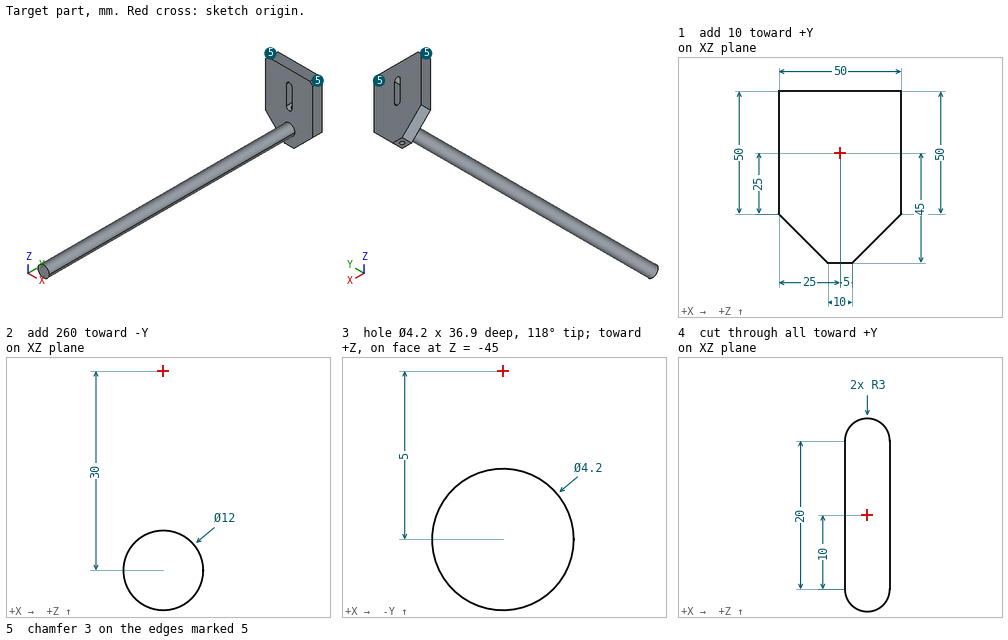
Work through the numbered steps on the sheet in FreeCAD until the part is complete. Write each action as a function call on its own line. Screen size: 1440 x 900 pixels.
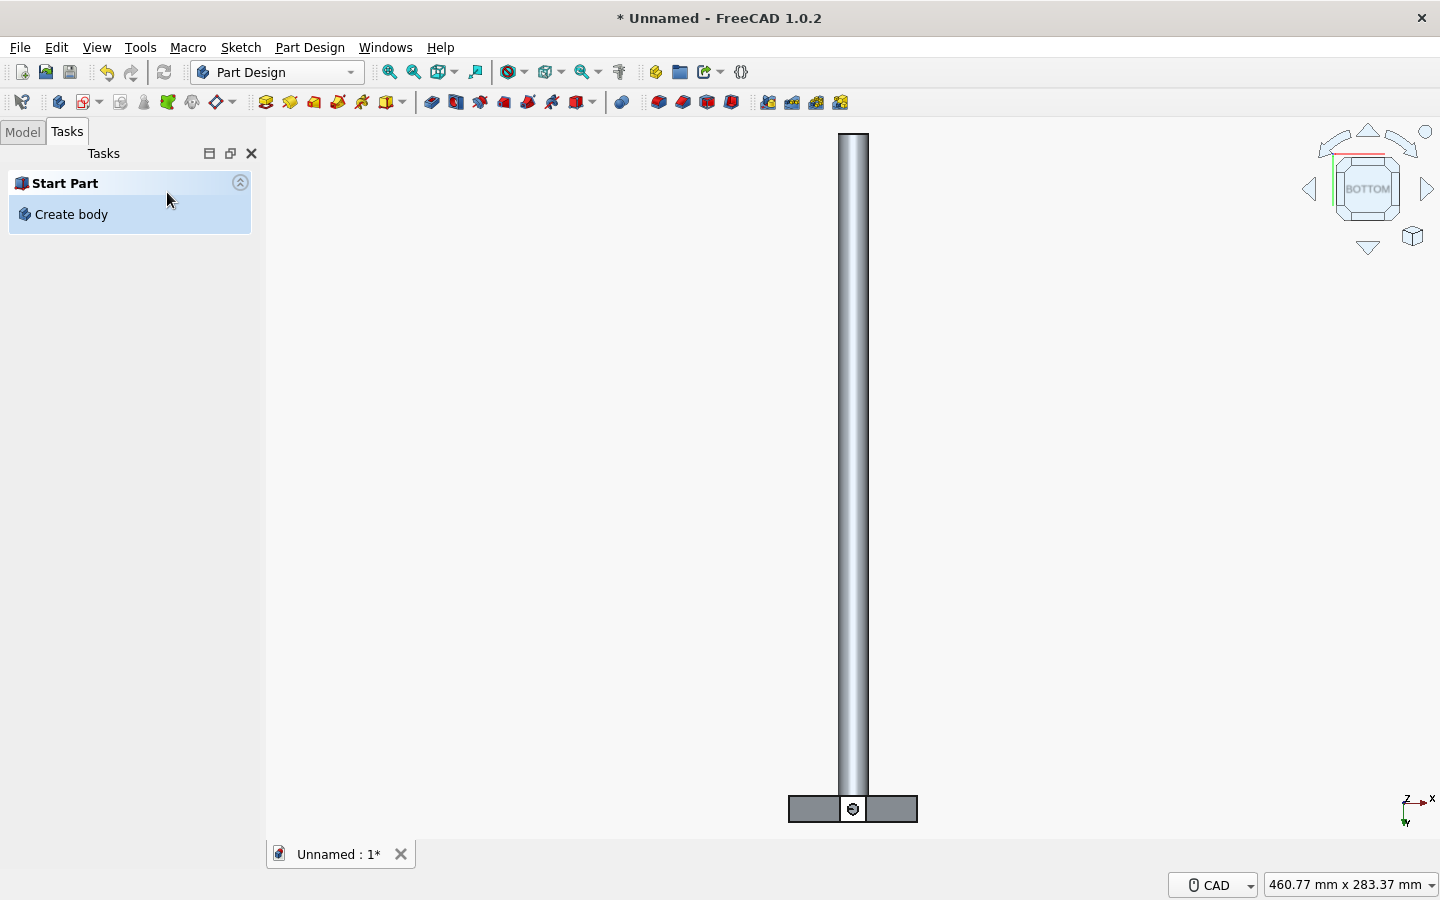
click(84, 102)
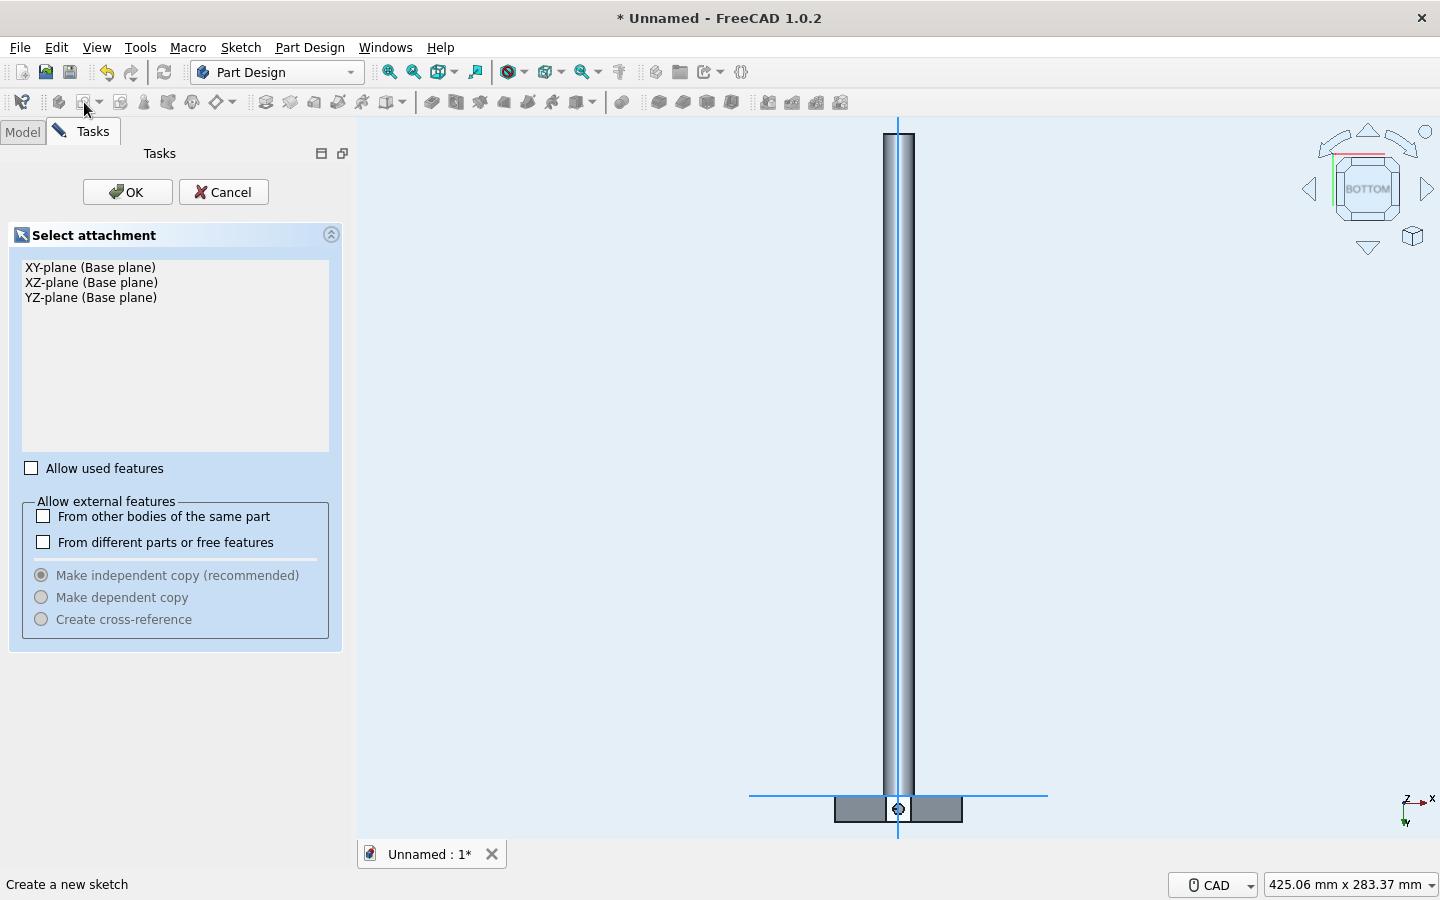
click(82, 282)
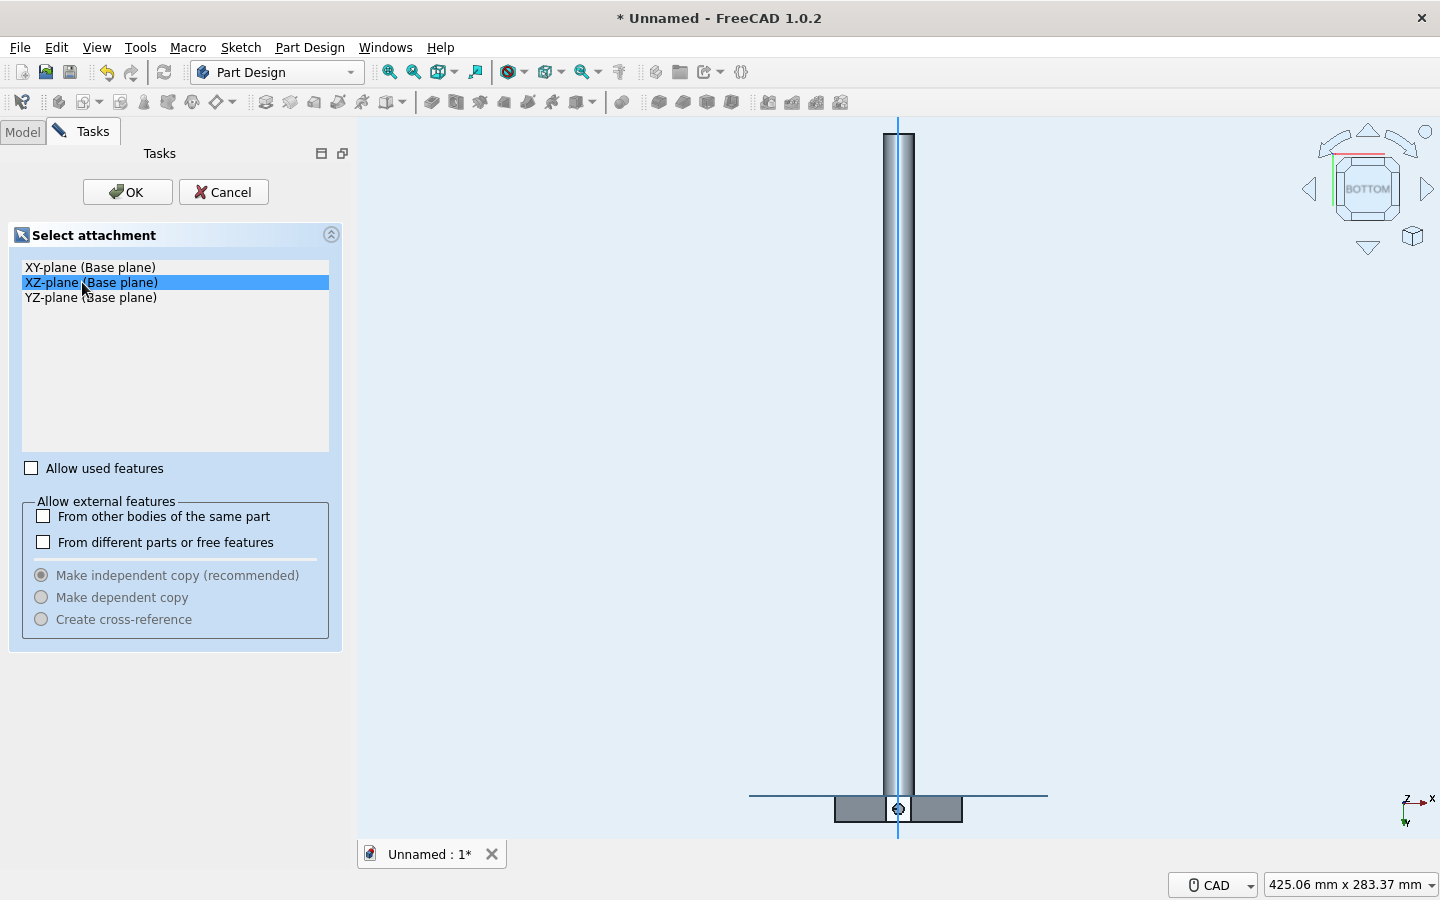
click(128, 192)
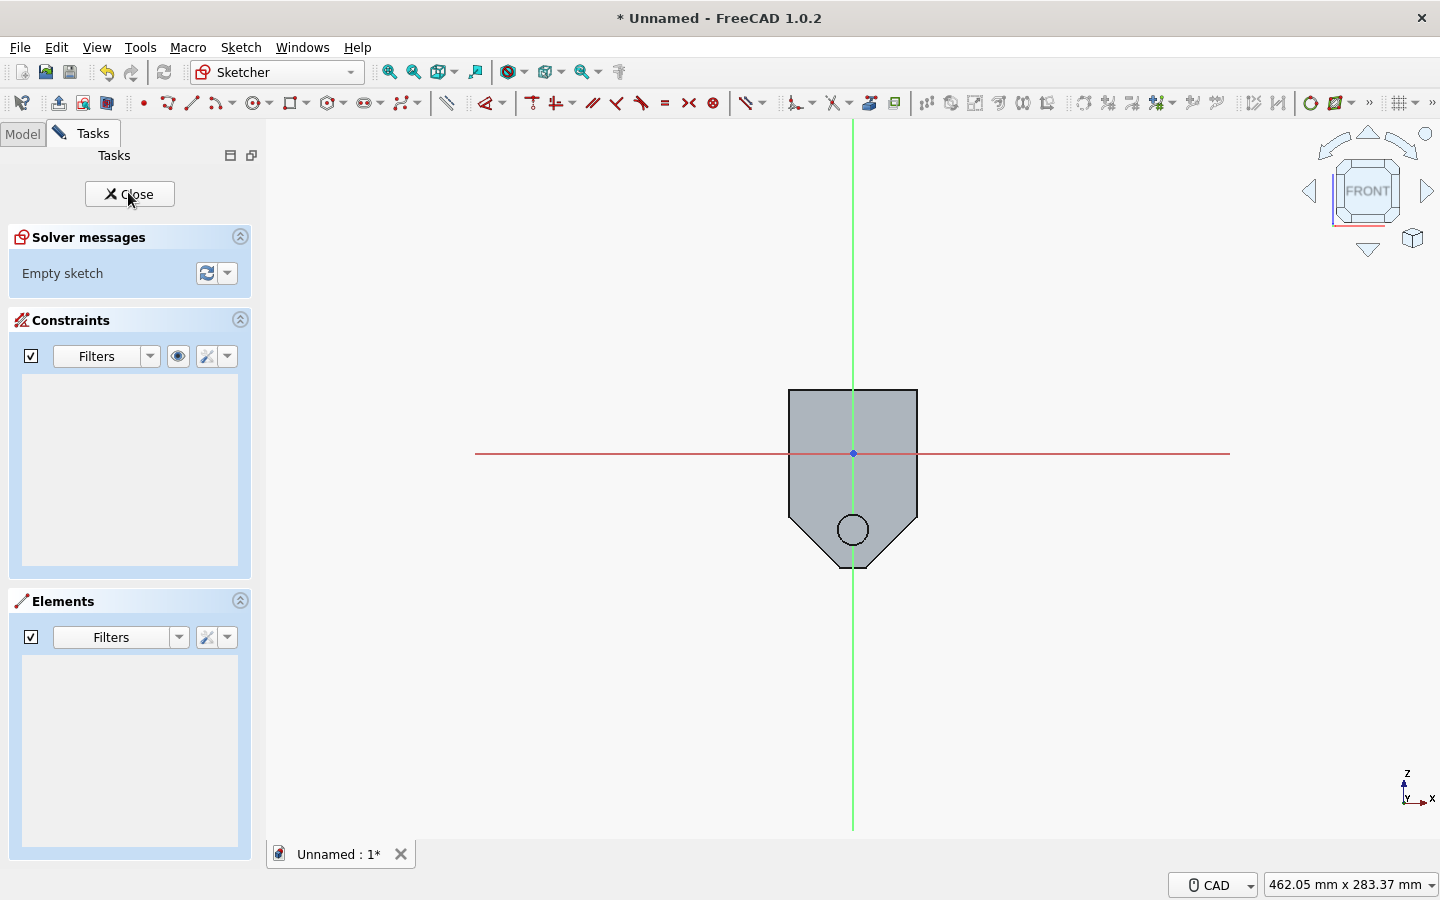
click(108, 104)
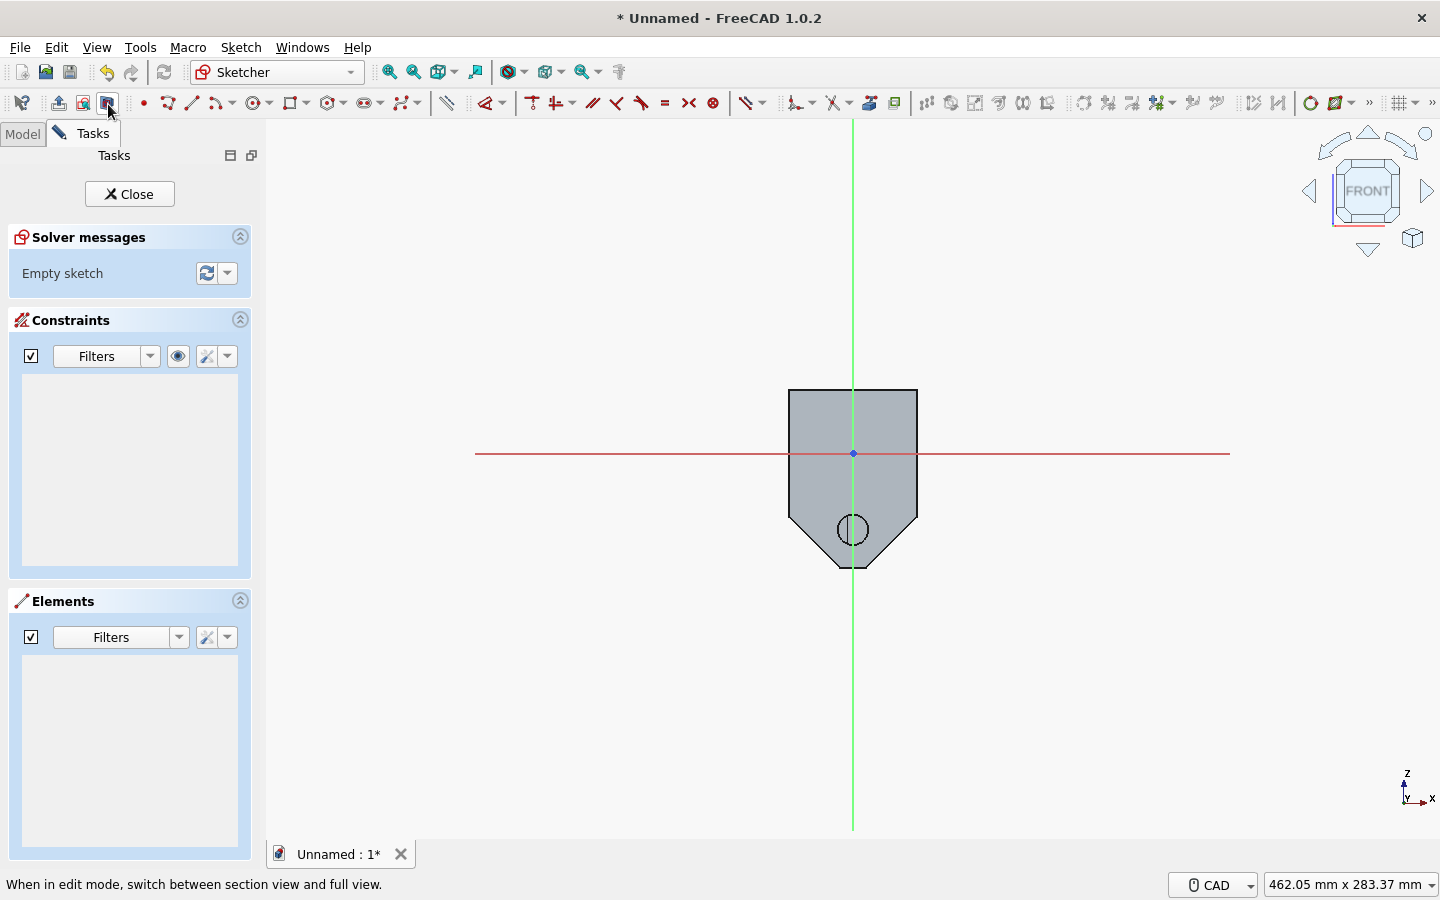
scroll(864, 450, up, 10)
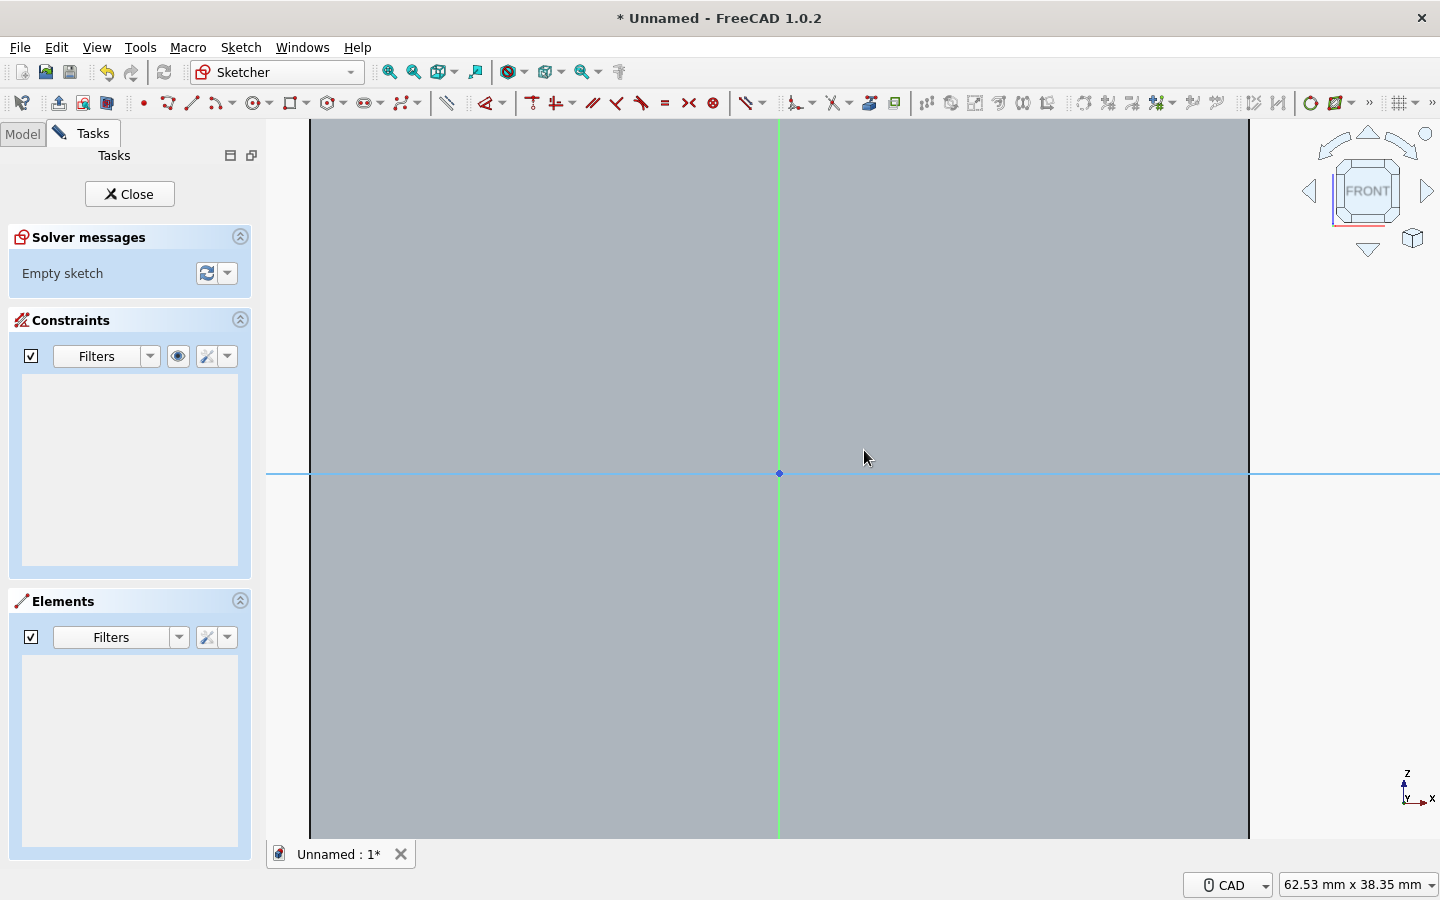
click(364, 104)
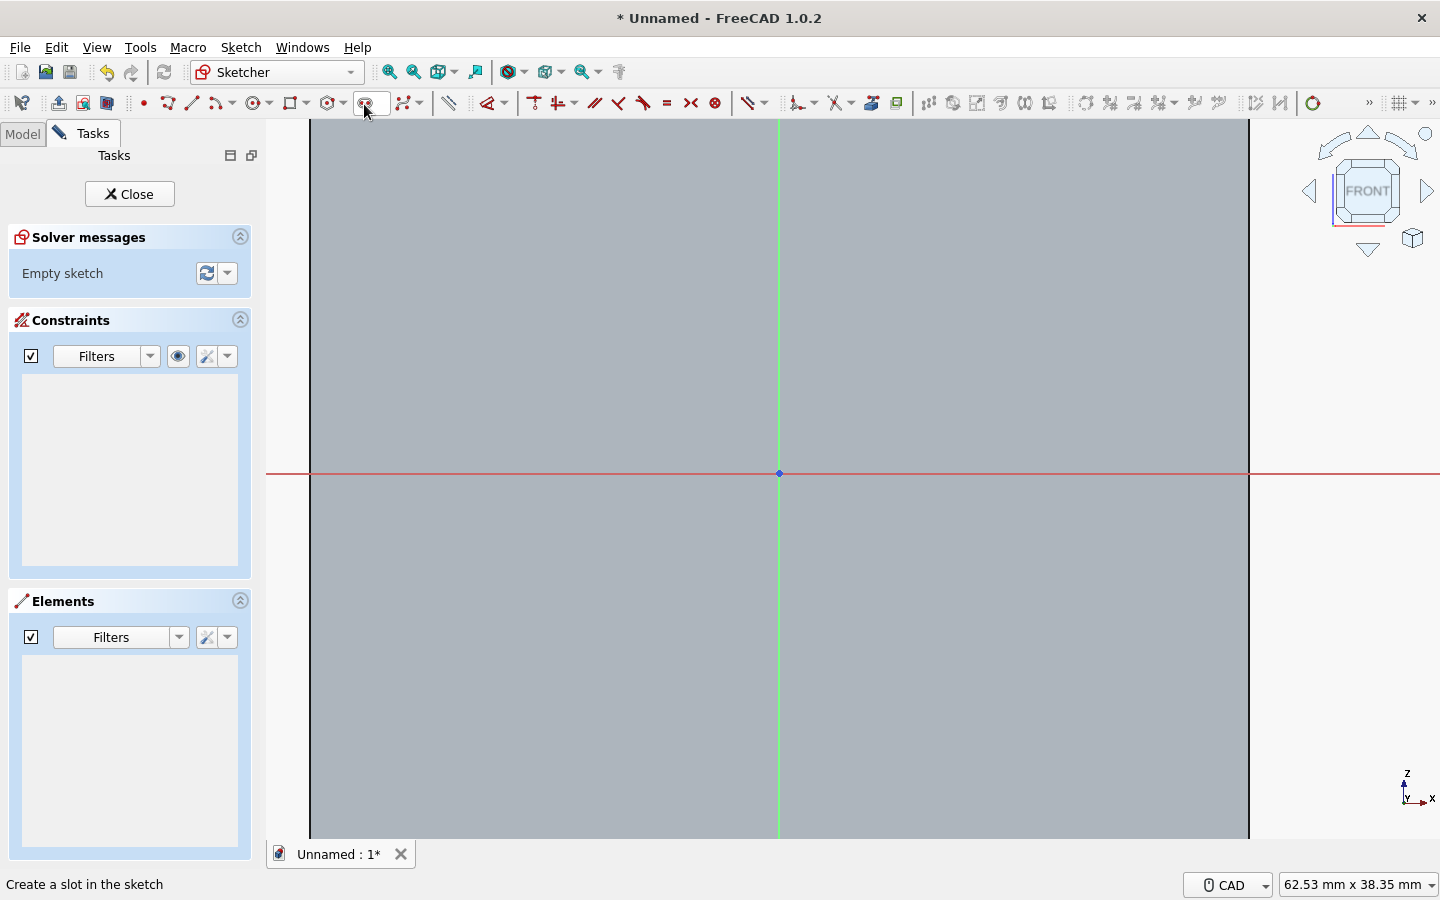
click(779, 661)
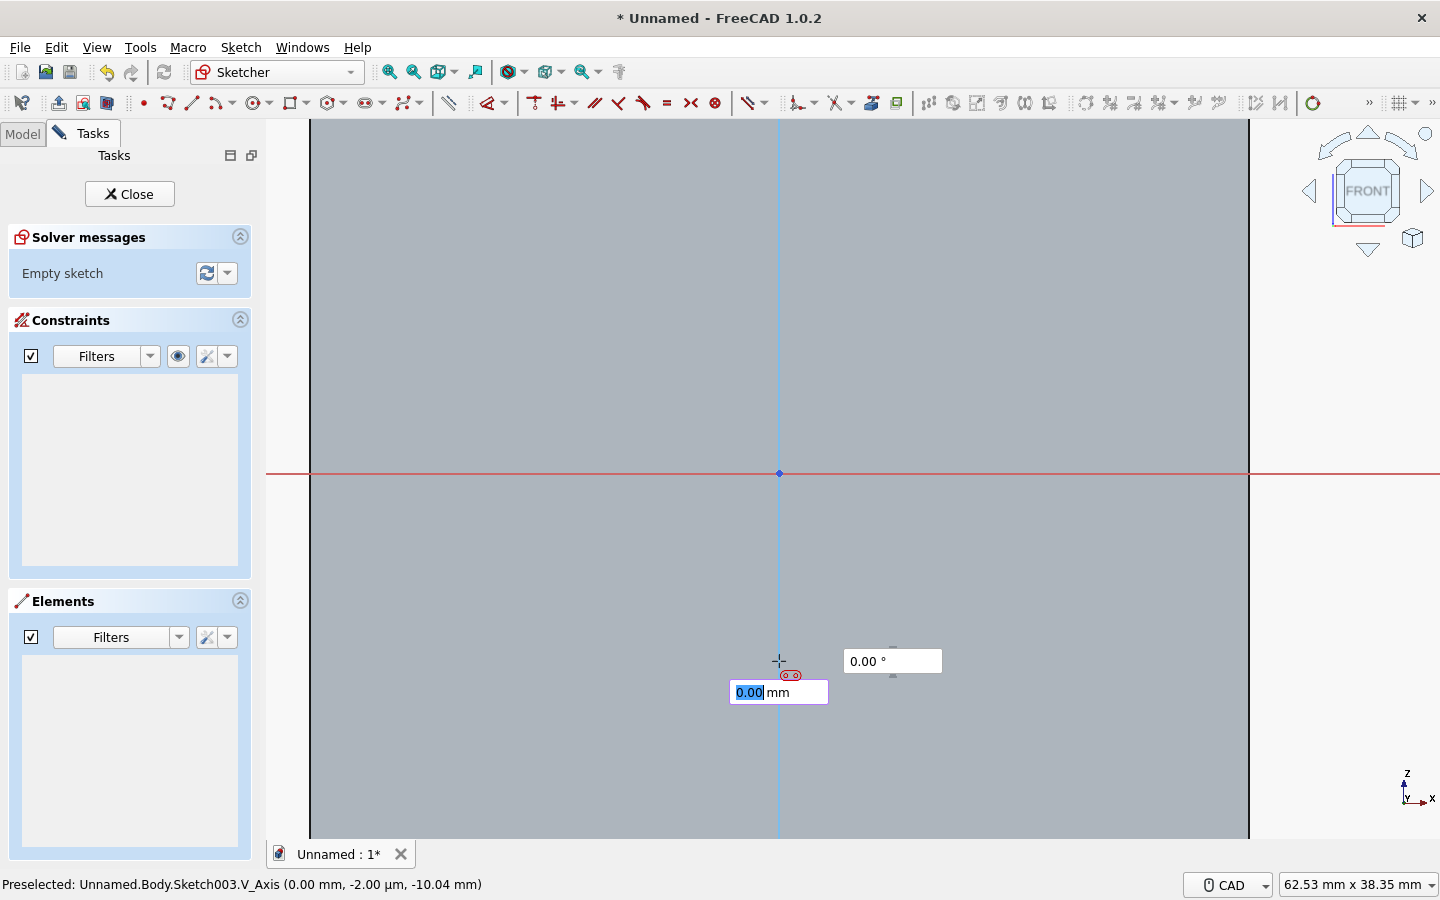
click(788, 286)